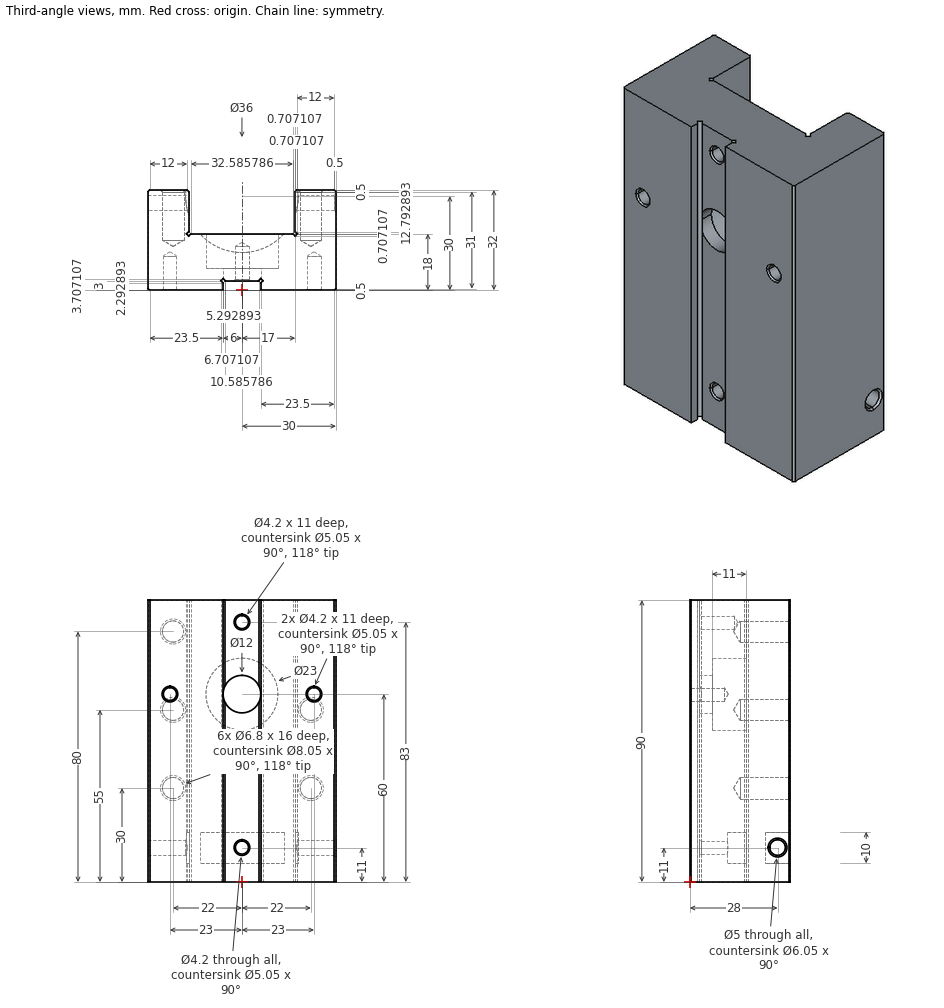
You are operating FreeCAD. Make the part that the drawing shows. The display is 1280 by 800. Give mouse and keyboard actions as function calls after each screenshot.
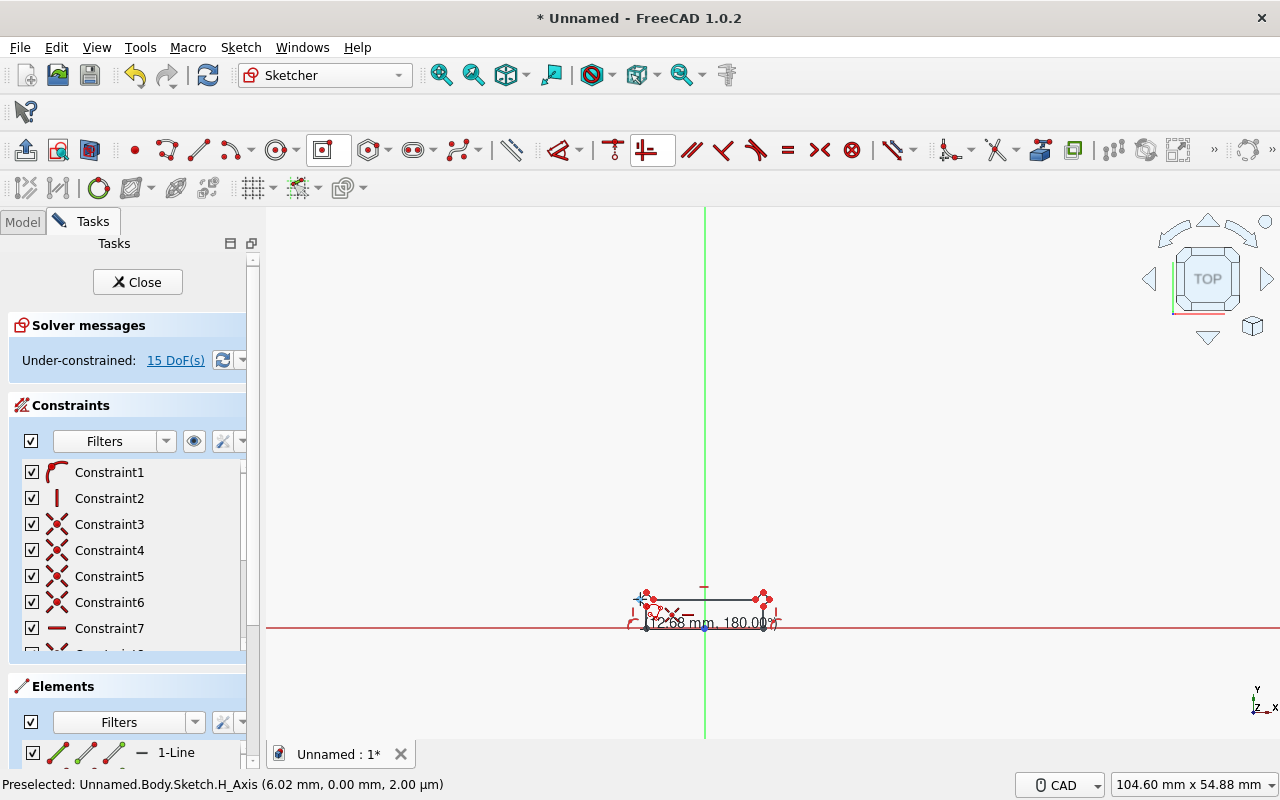
click(991, 619)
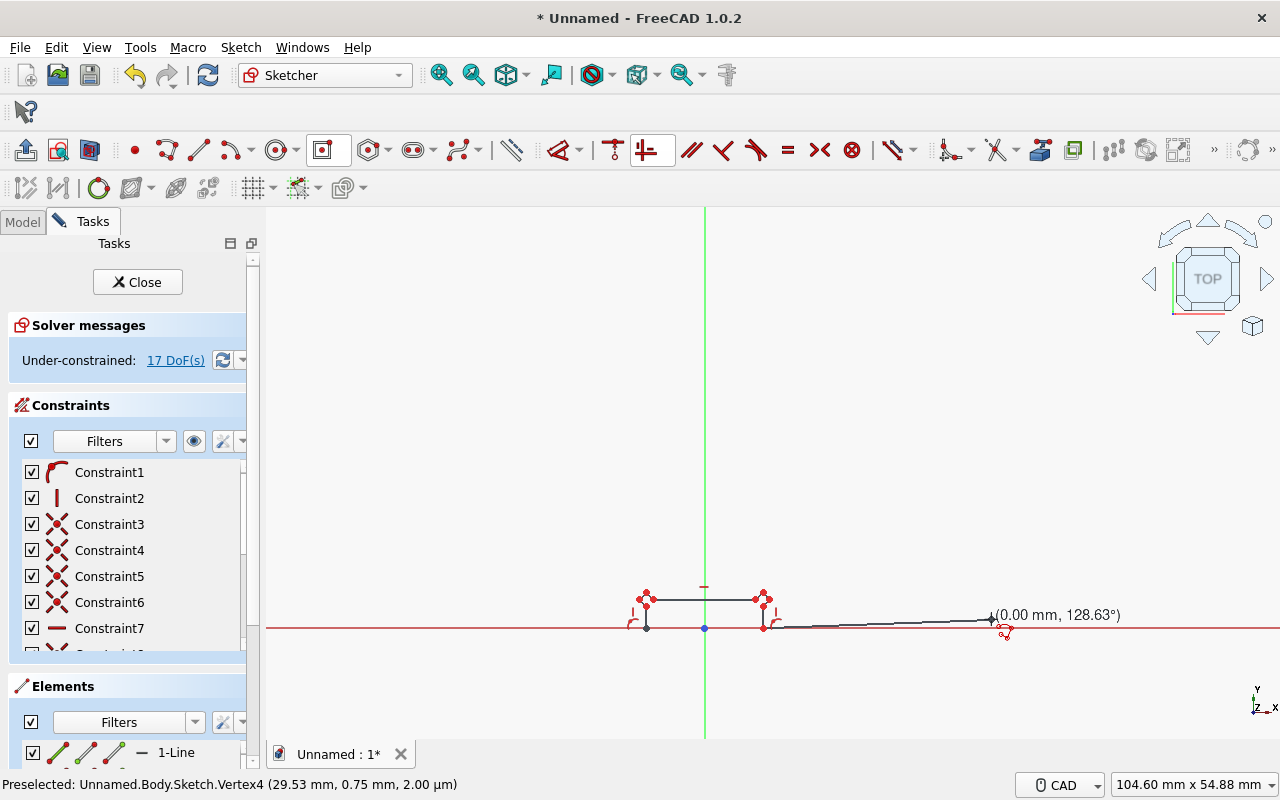
scroll(996, 623, up, 6)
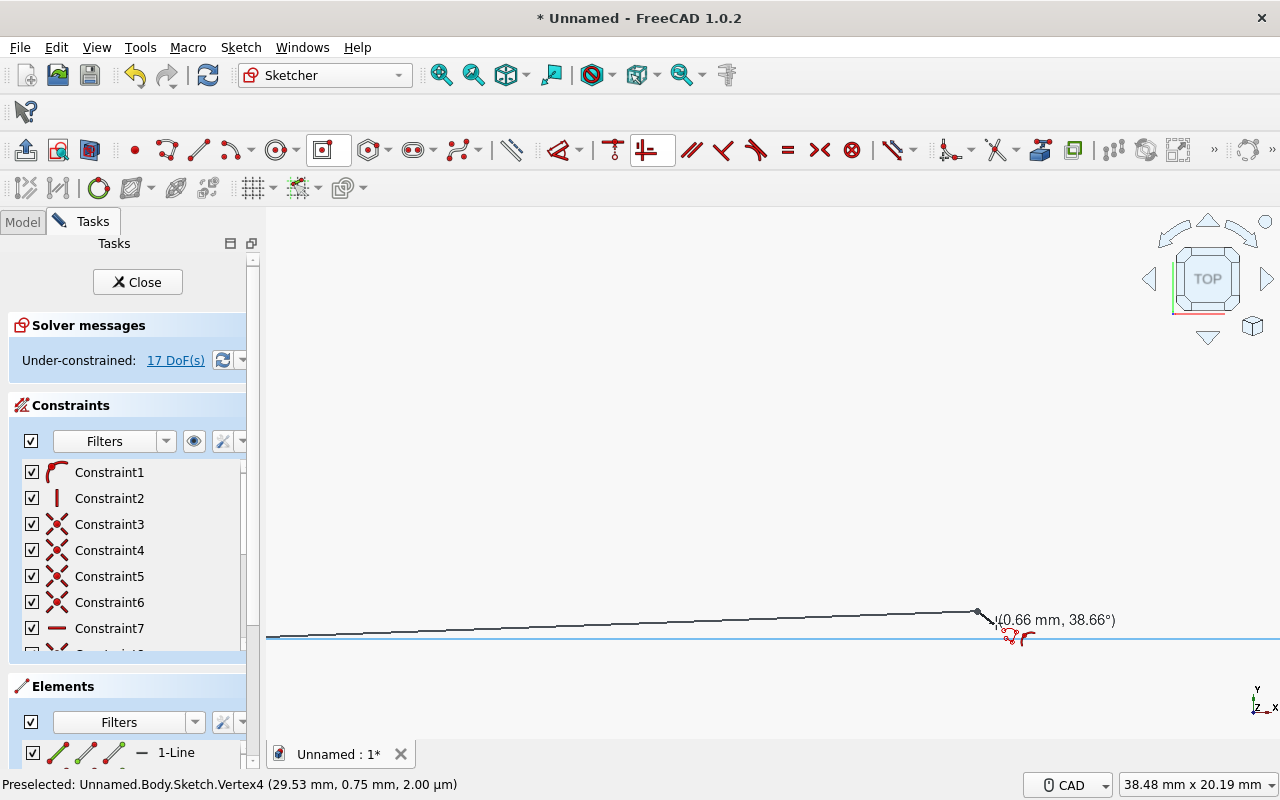
click(993, 623)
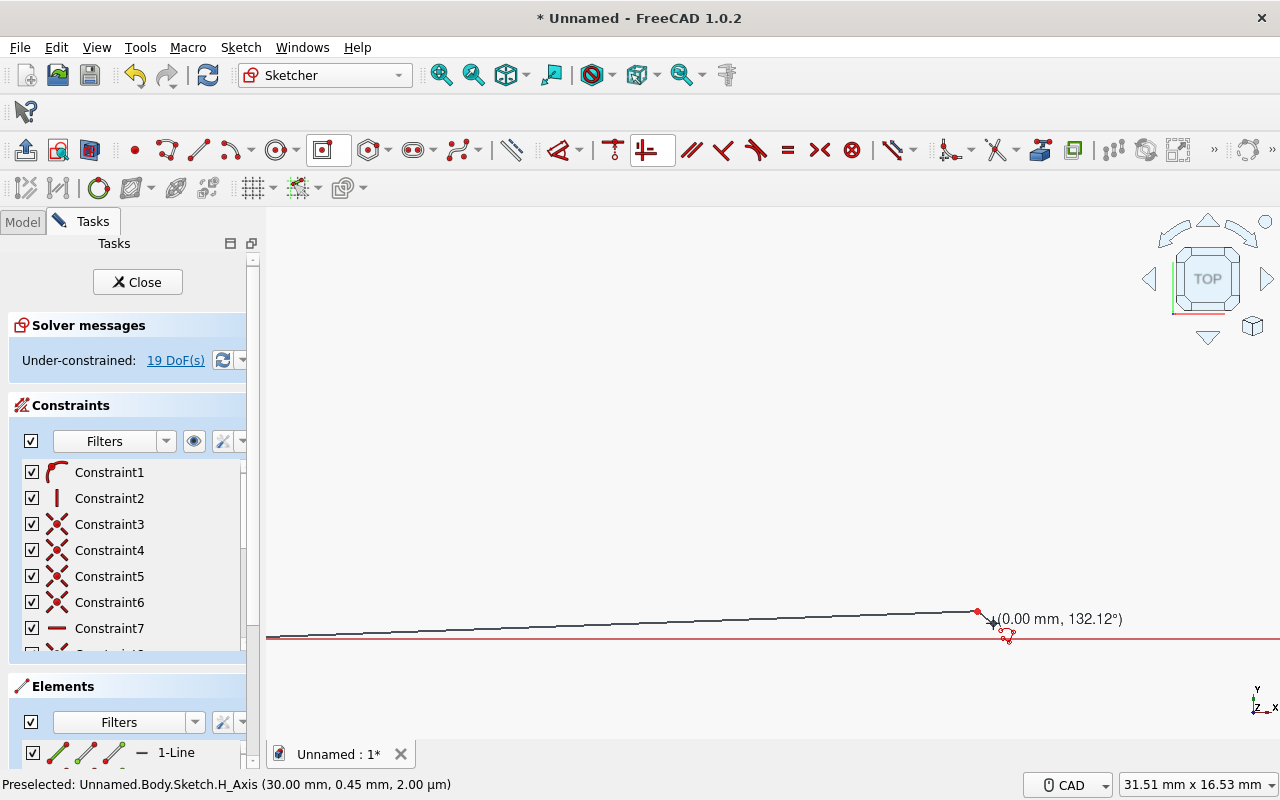
scroll(996, 624, down, 6)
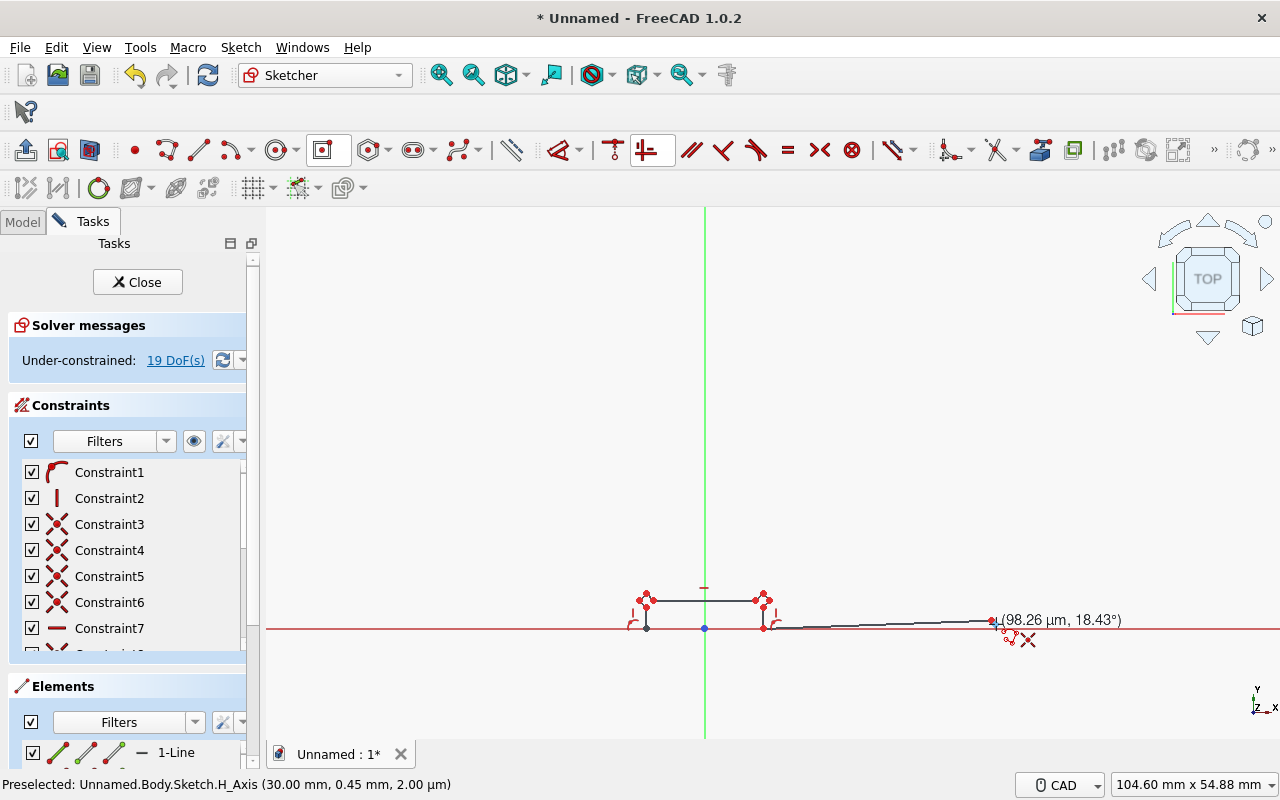
click(996, 324)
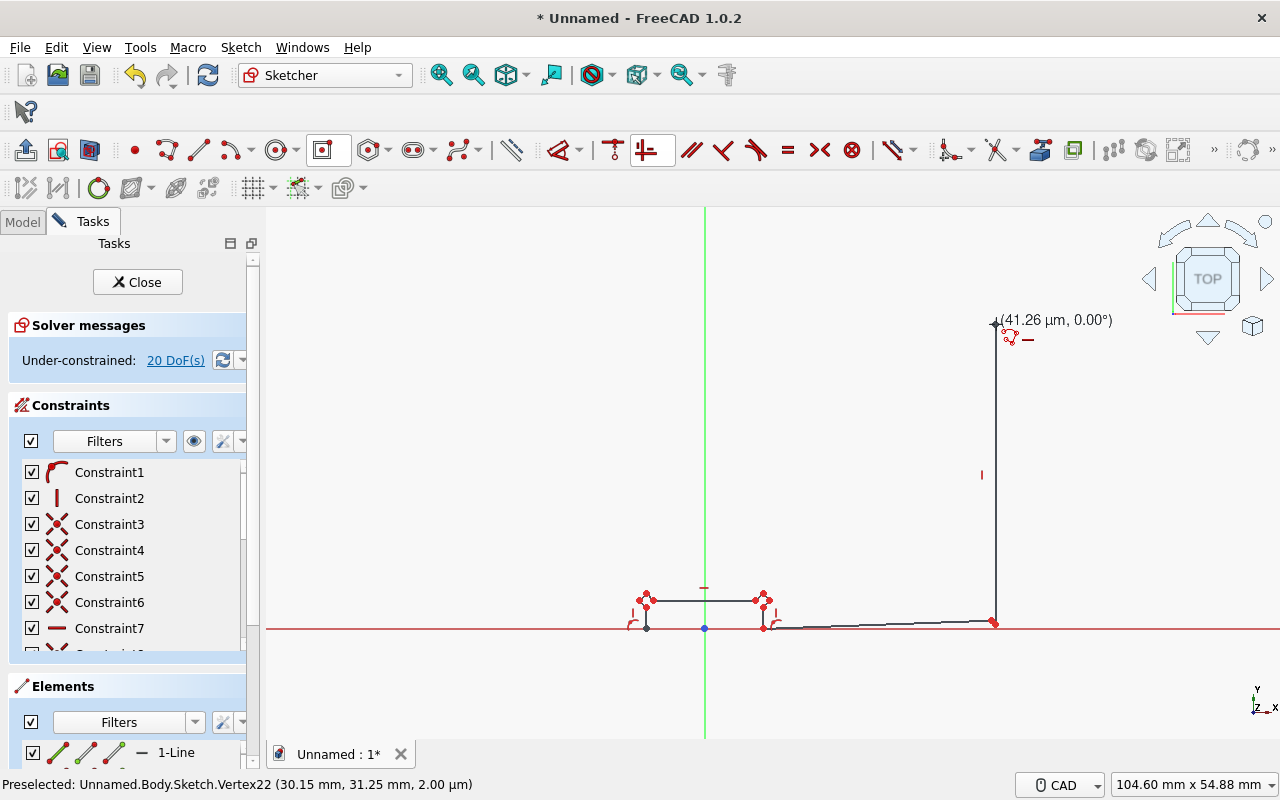
scroll(991, 319, up, 5)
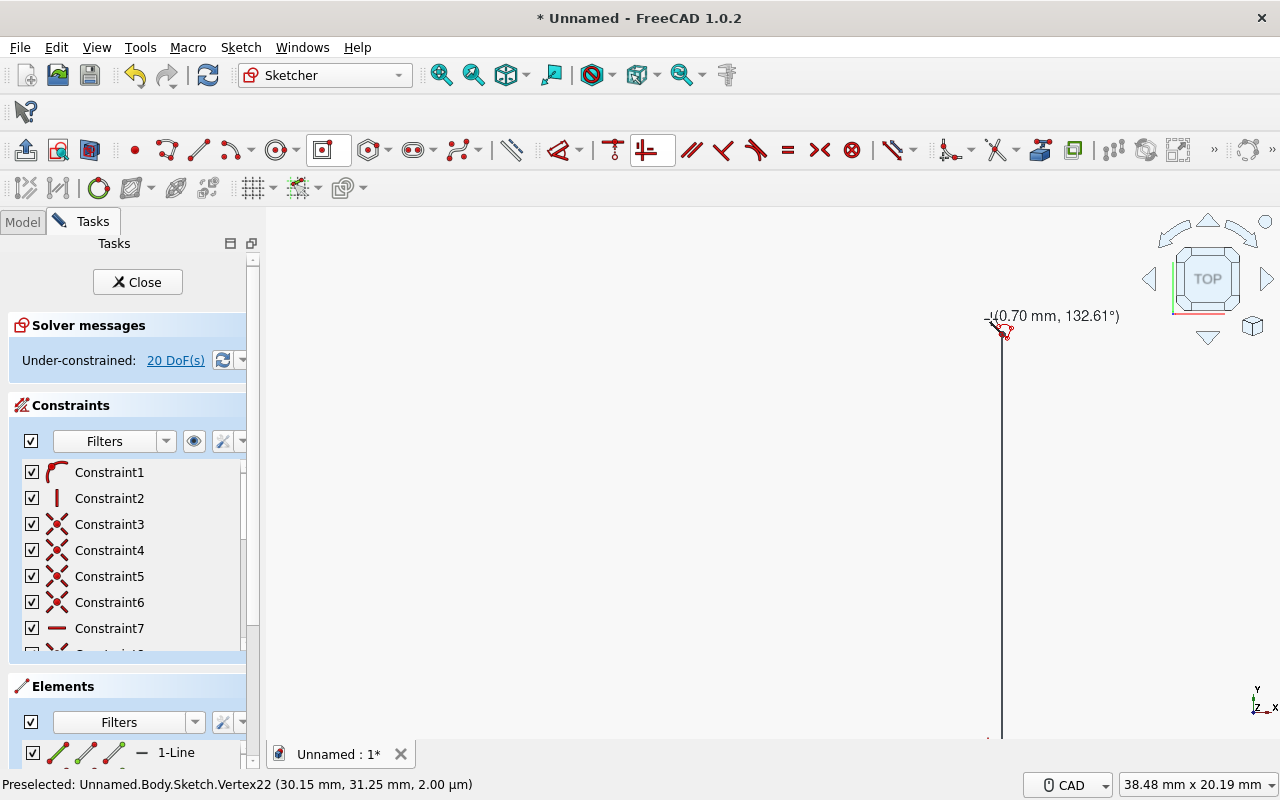
click(989, 318)
click(673, 318)
click(660, 331)
click(660, 668)
click(678, 687)
click(660, 706)
click(641, 687)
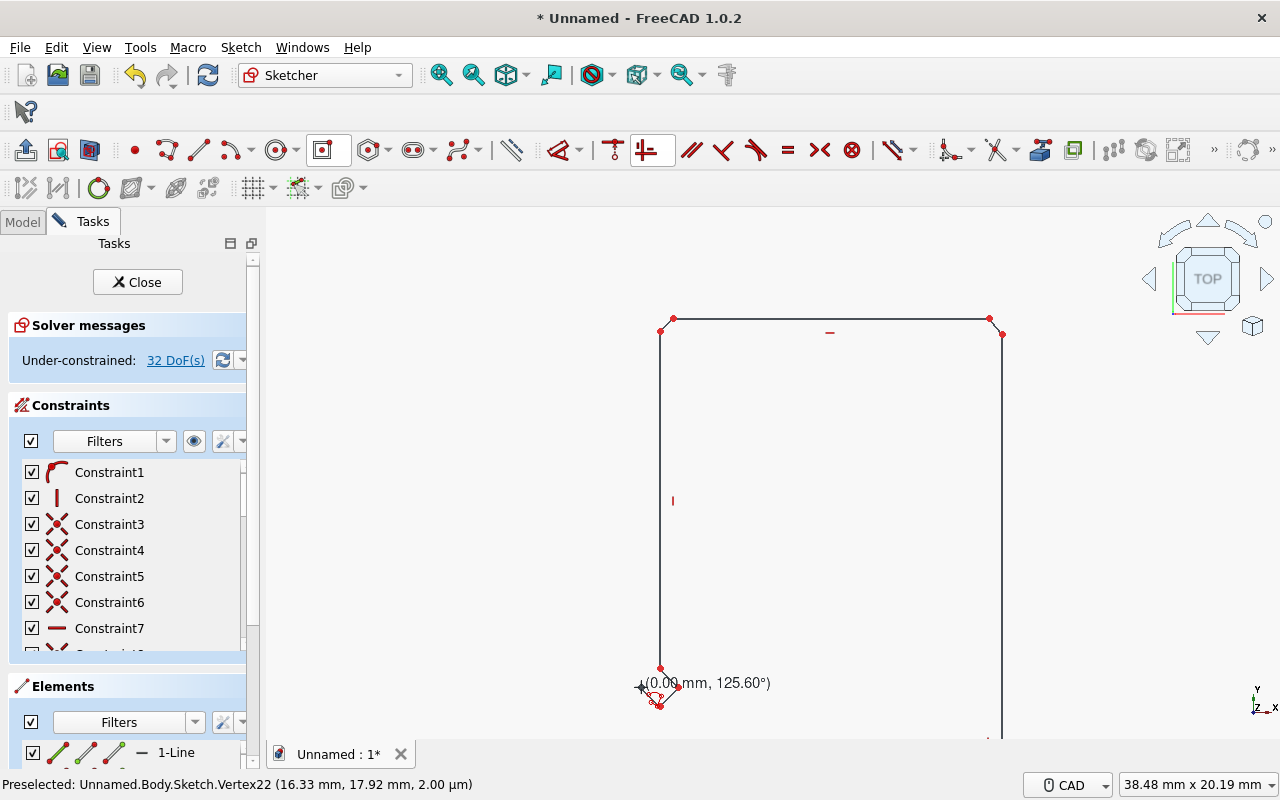
scroll(991, 318, down, 5)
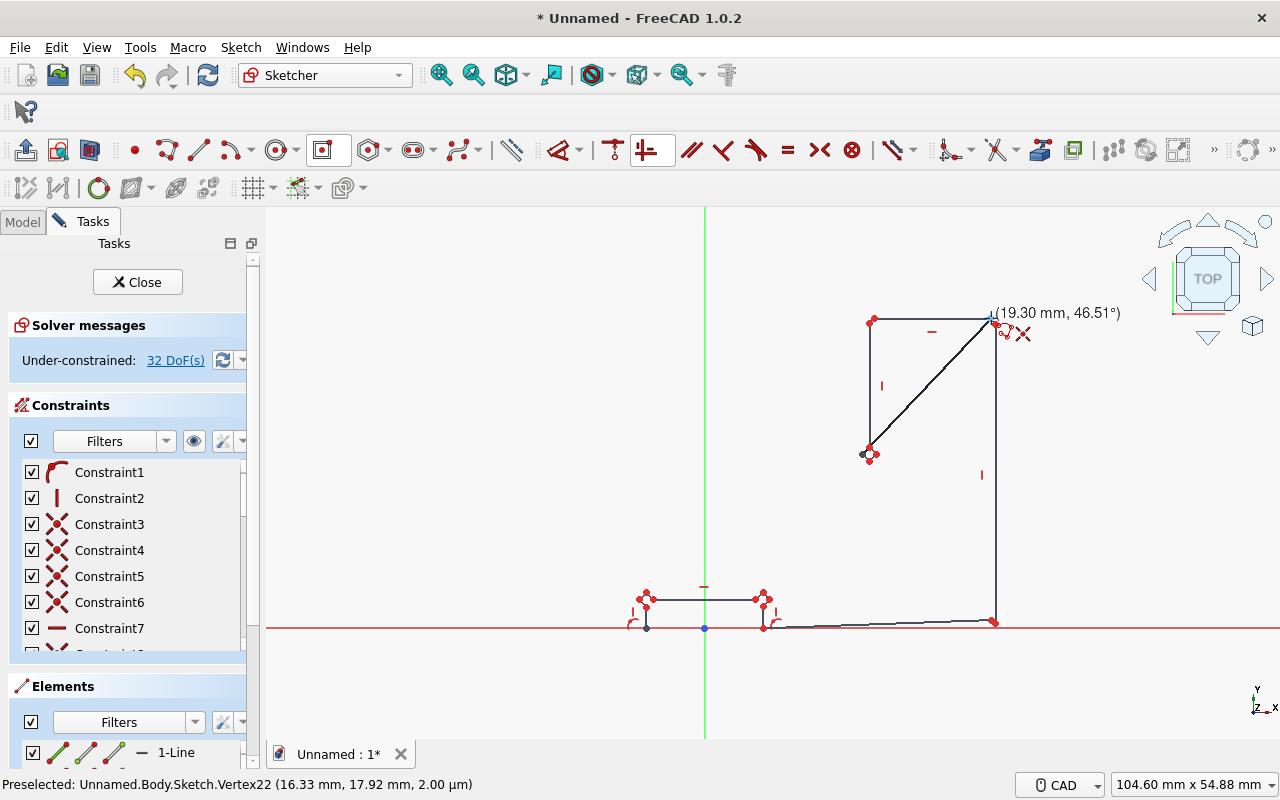
click(547, 454)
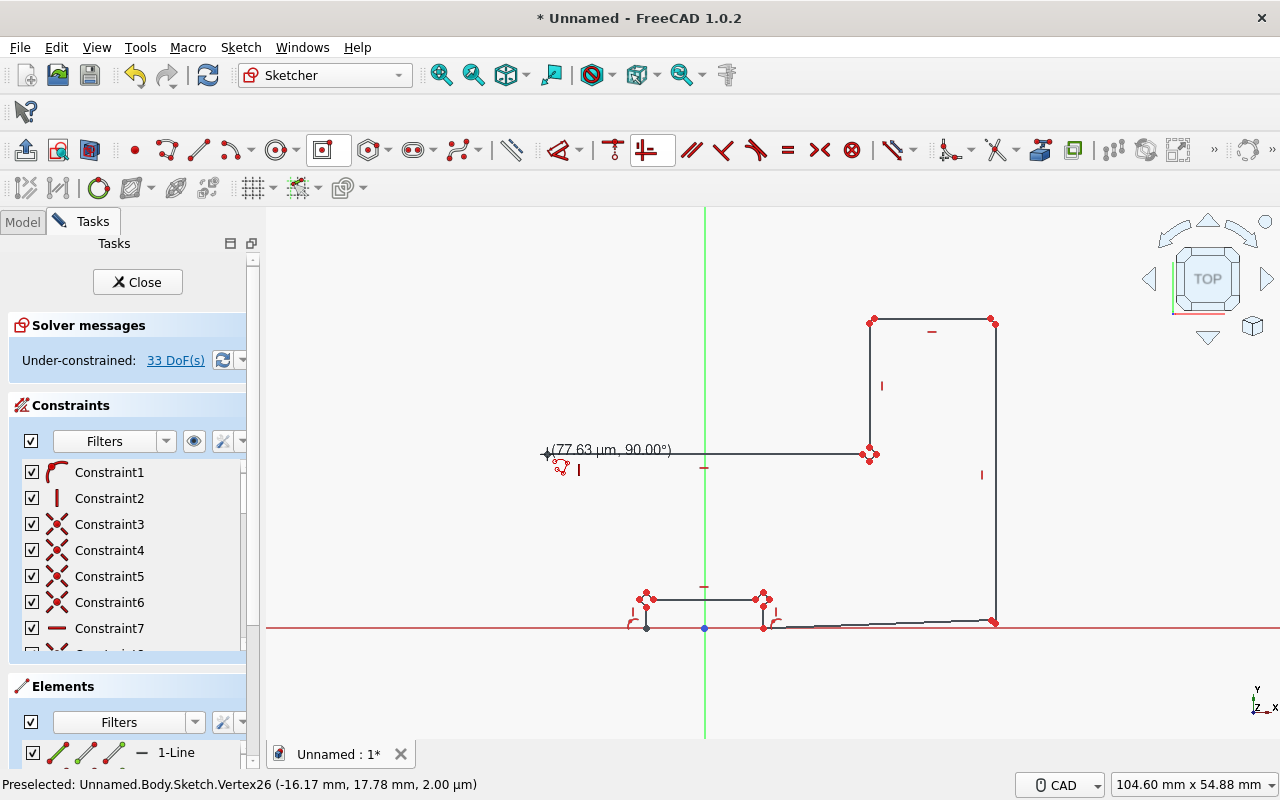
scroll(540, 461, up, 3)